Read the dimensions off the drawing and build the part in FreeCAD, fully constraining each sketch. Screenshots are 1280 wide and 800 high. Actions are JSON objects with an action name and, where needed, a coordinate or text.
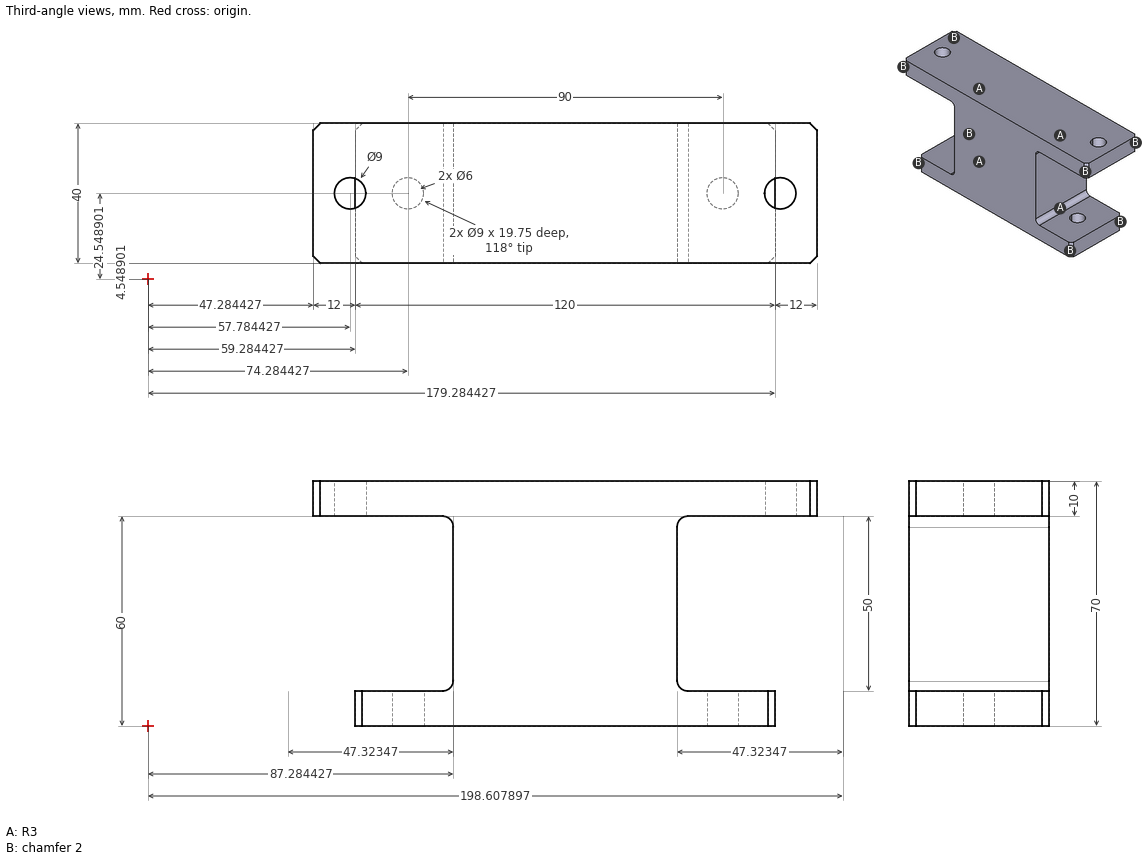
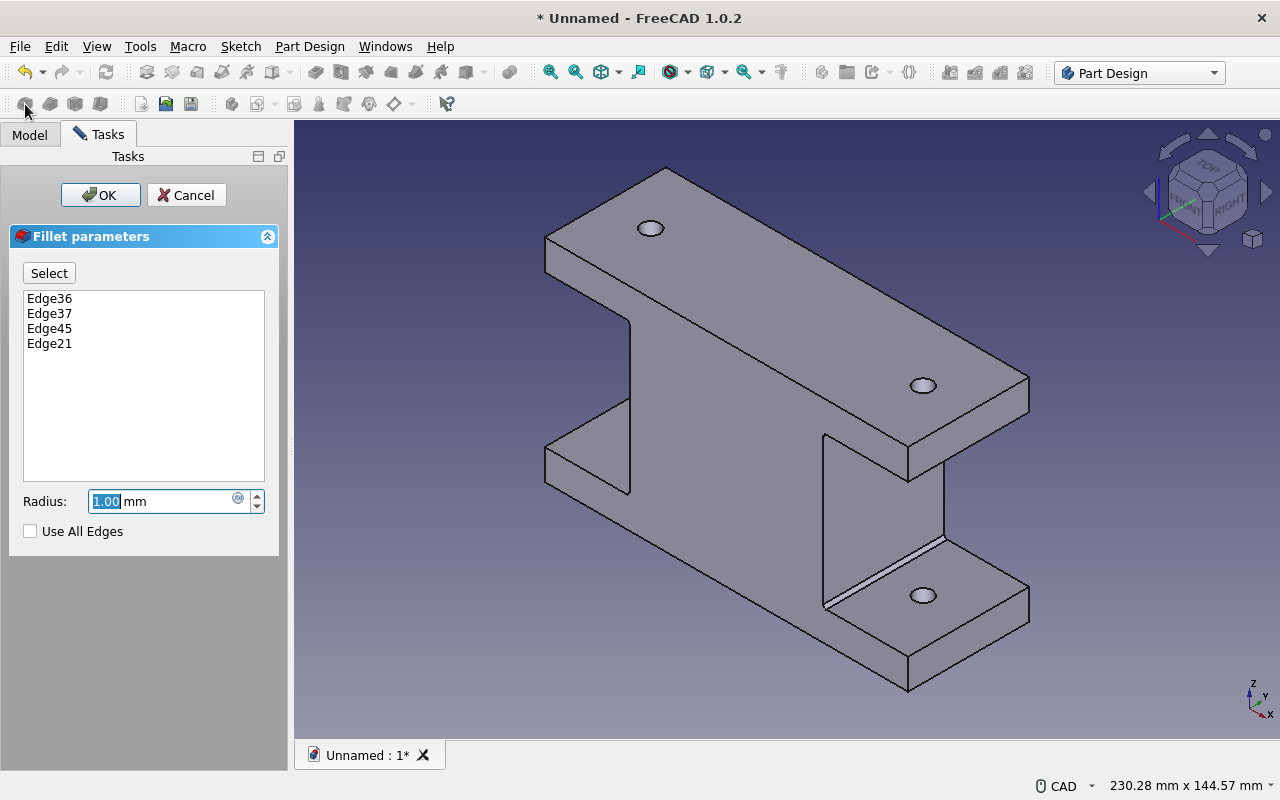
{"action": "type", "text": "3"}
{"action": "key", "text": "Tab"}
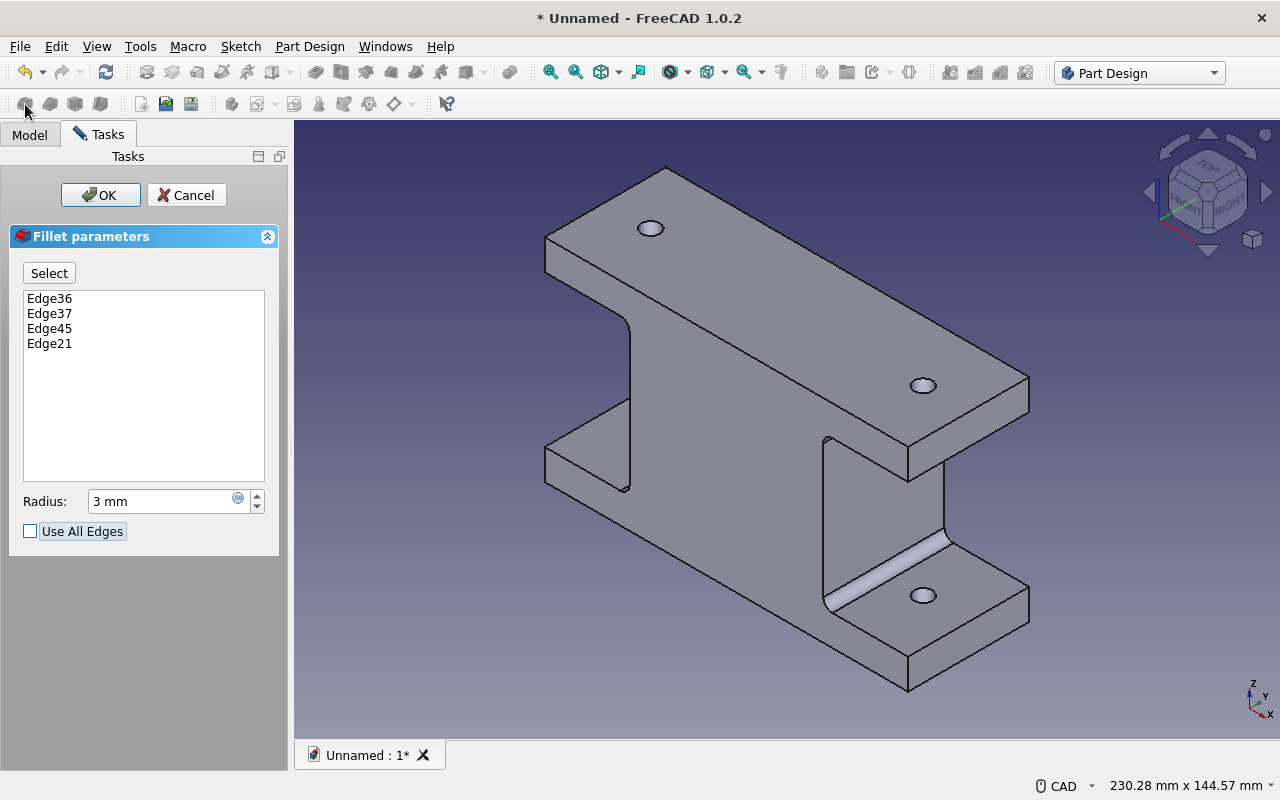
{"action": "left_click", "coordinate": [101, 195]}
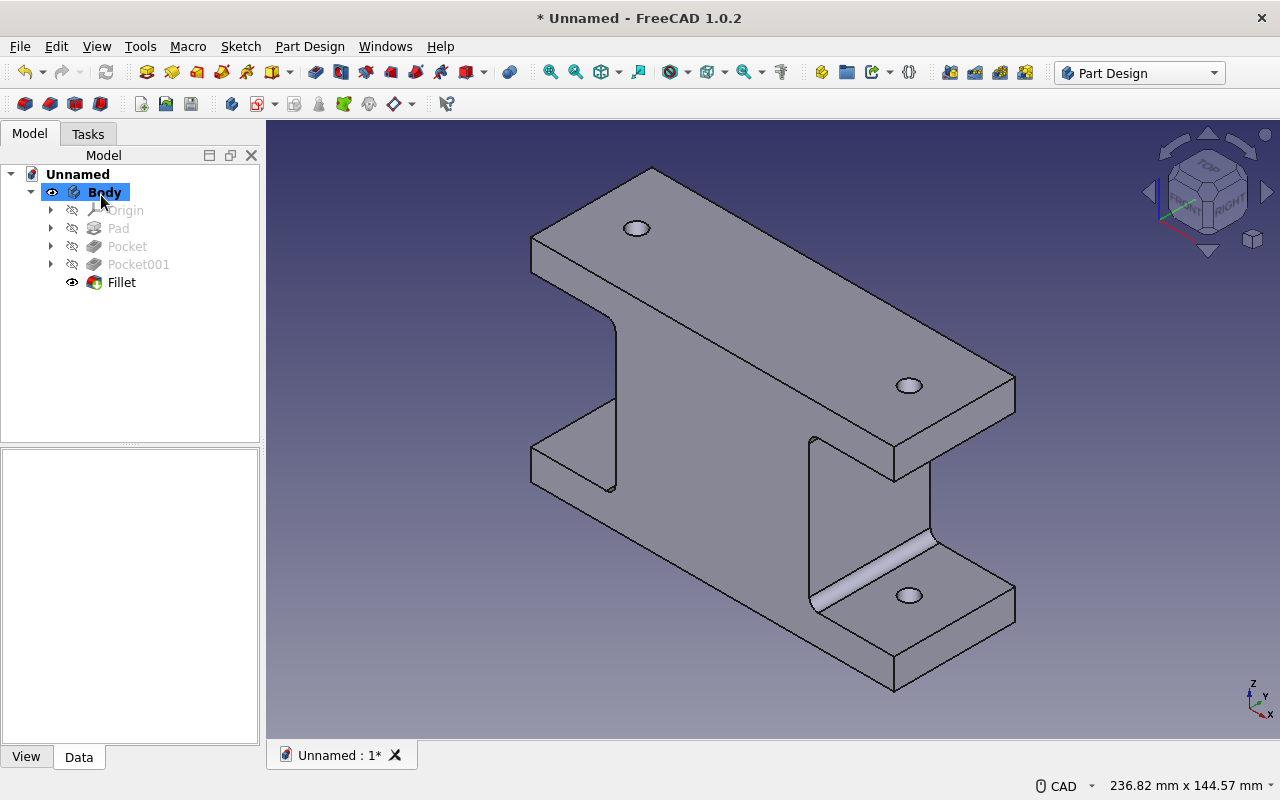
{"action": "left_click", "coordinate": [51, 210]}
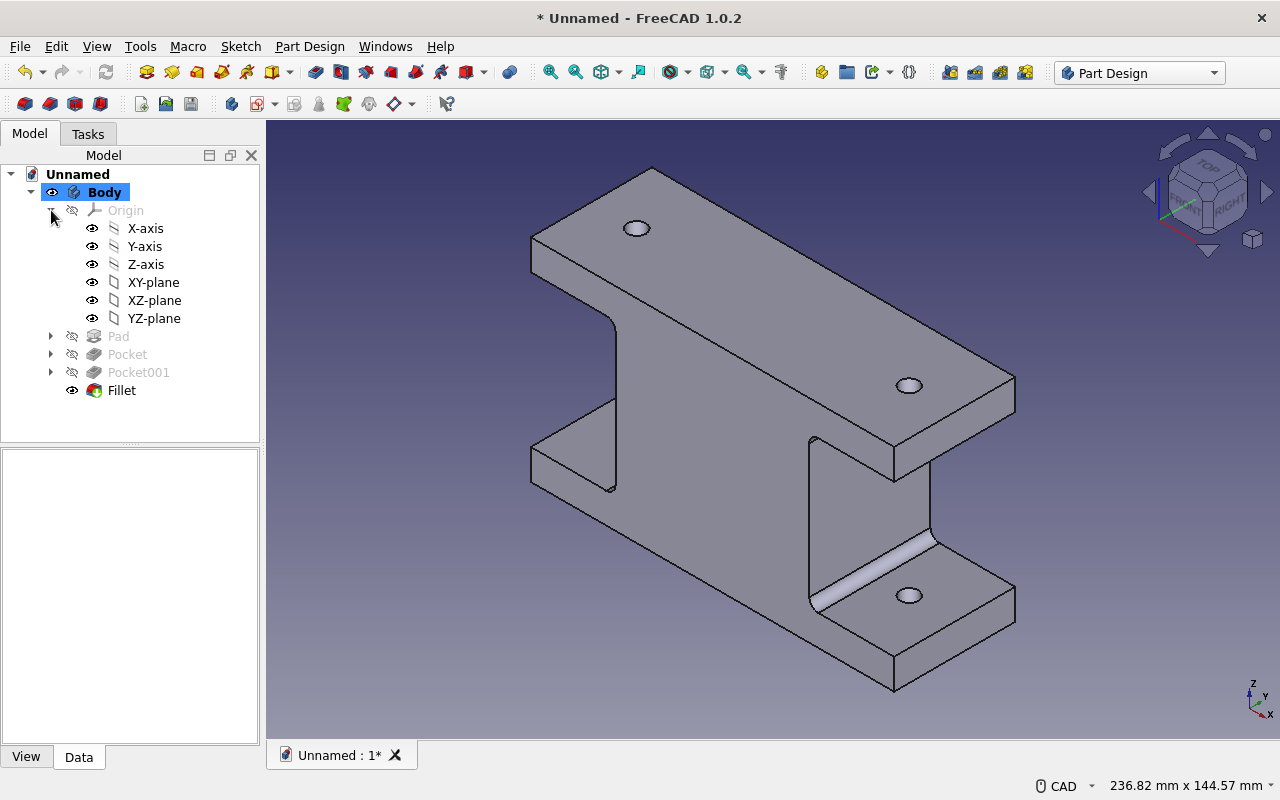
{"action": "left_click", "coordinate": [137, 282]}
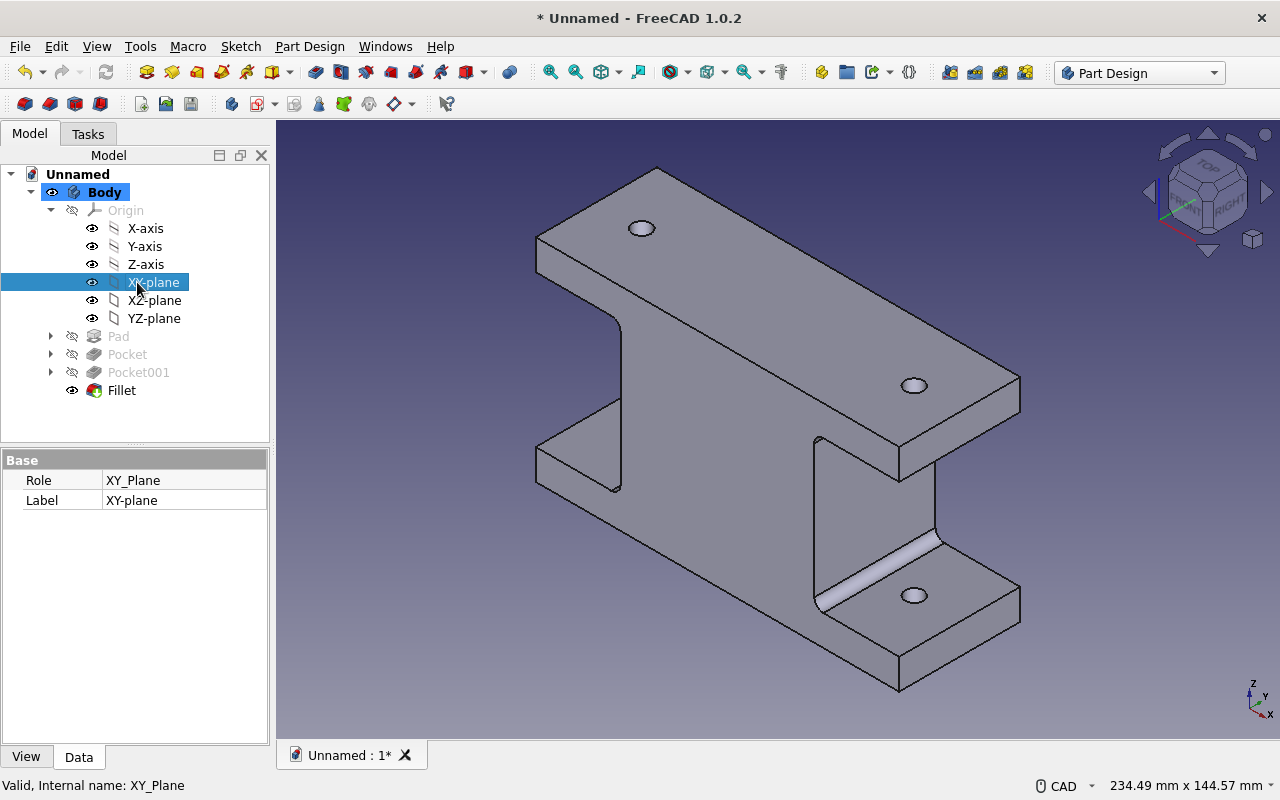
{"action": "left_click", "coordinate": [394, 104]}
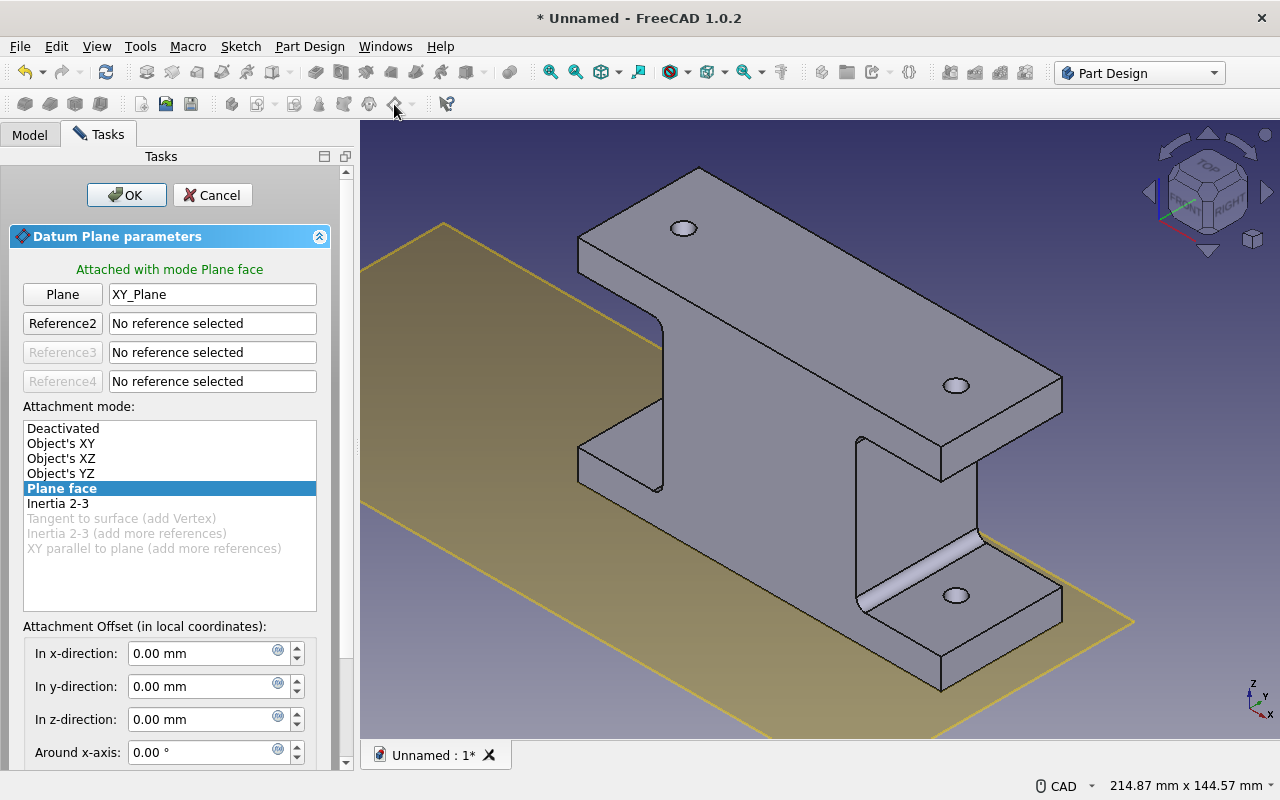
{"action": "triple_click", "coordinate": [210, 720]}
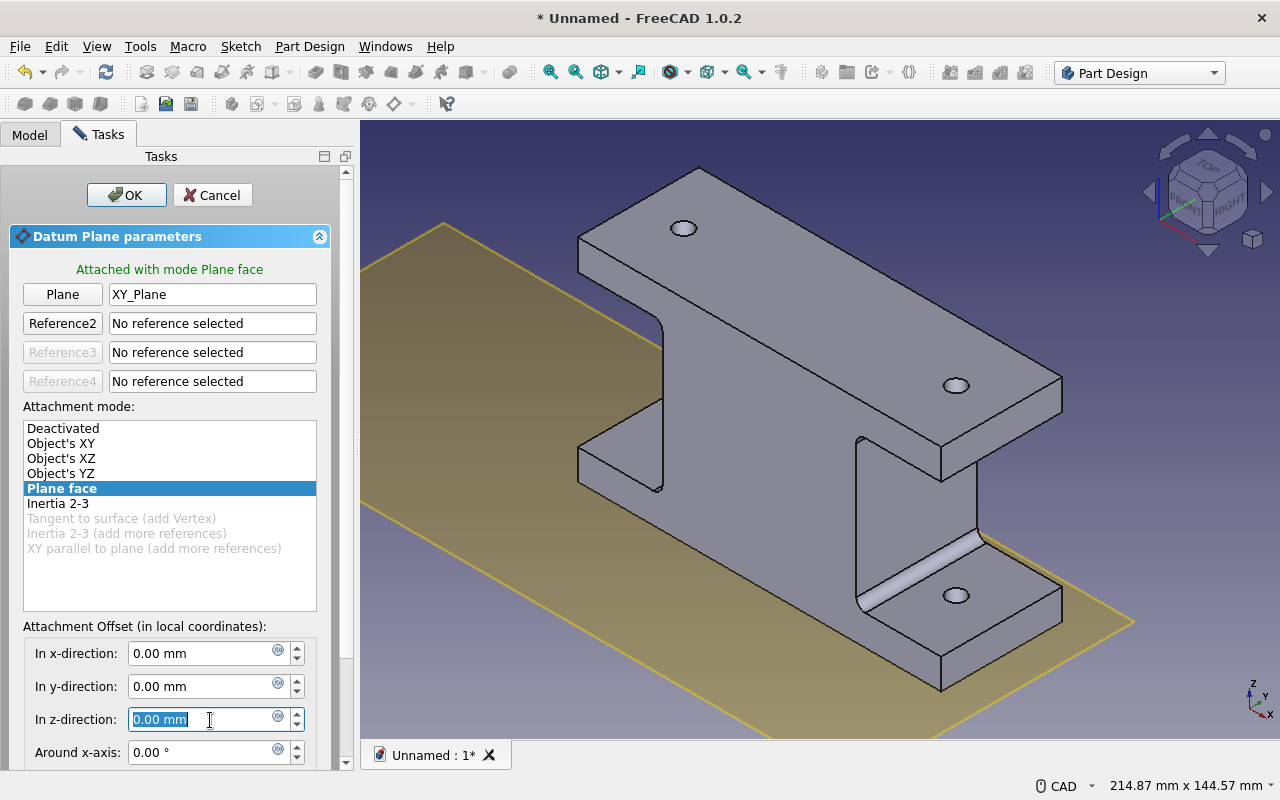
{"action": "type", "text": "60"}
{"action": "key", "text": "Tab"}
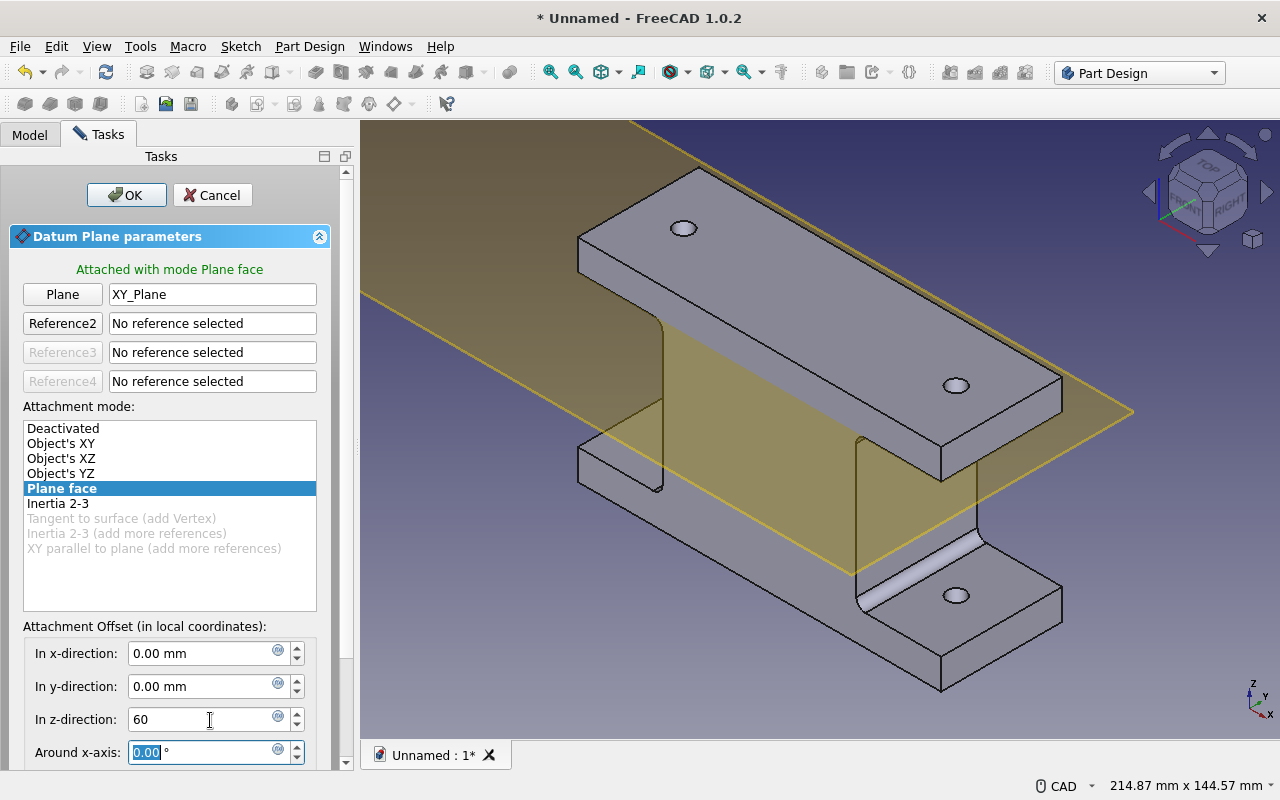
{"action": "left_click", "coordinate": [127, 195]}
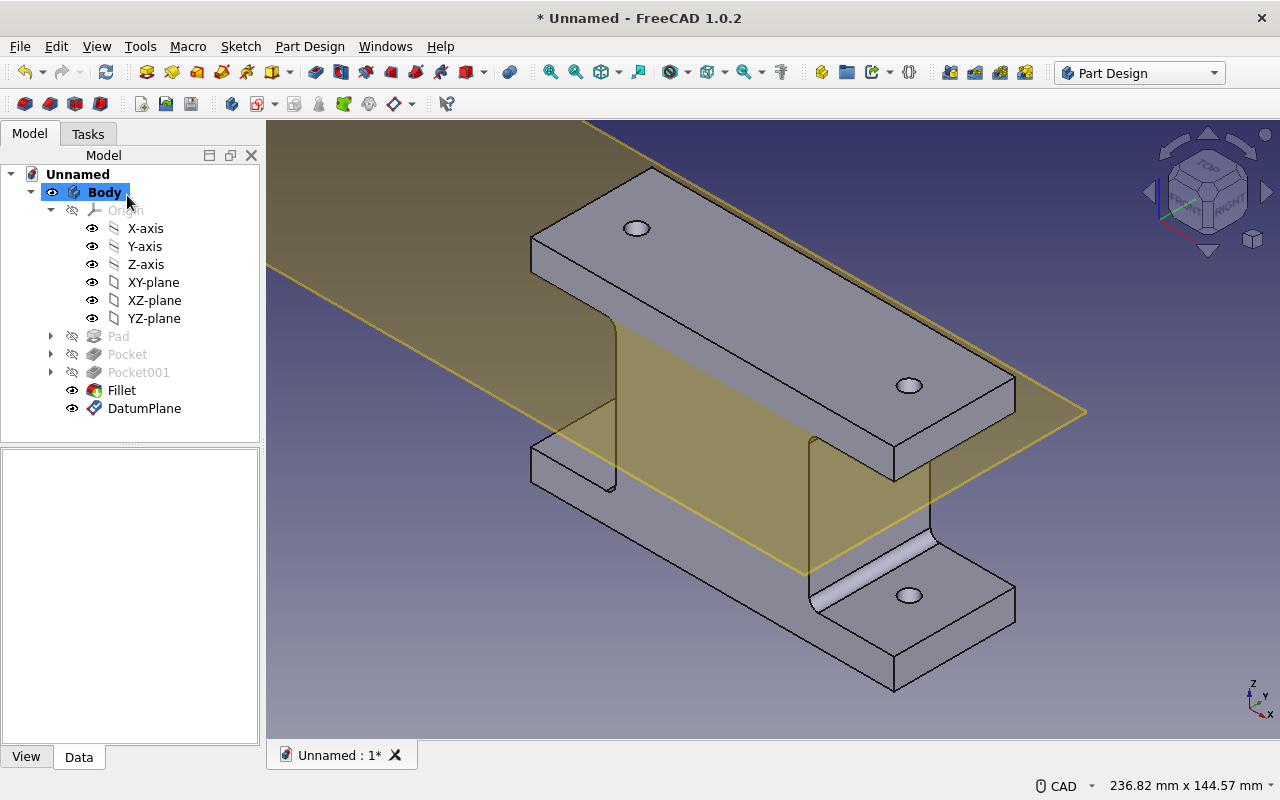
{"action": "left_click", "coordinate": [117, 408]}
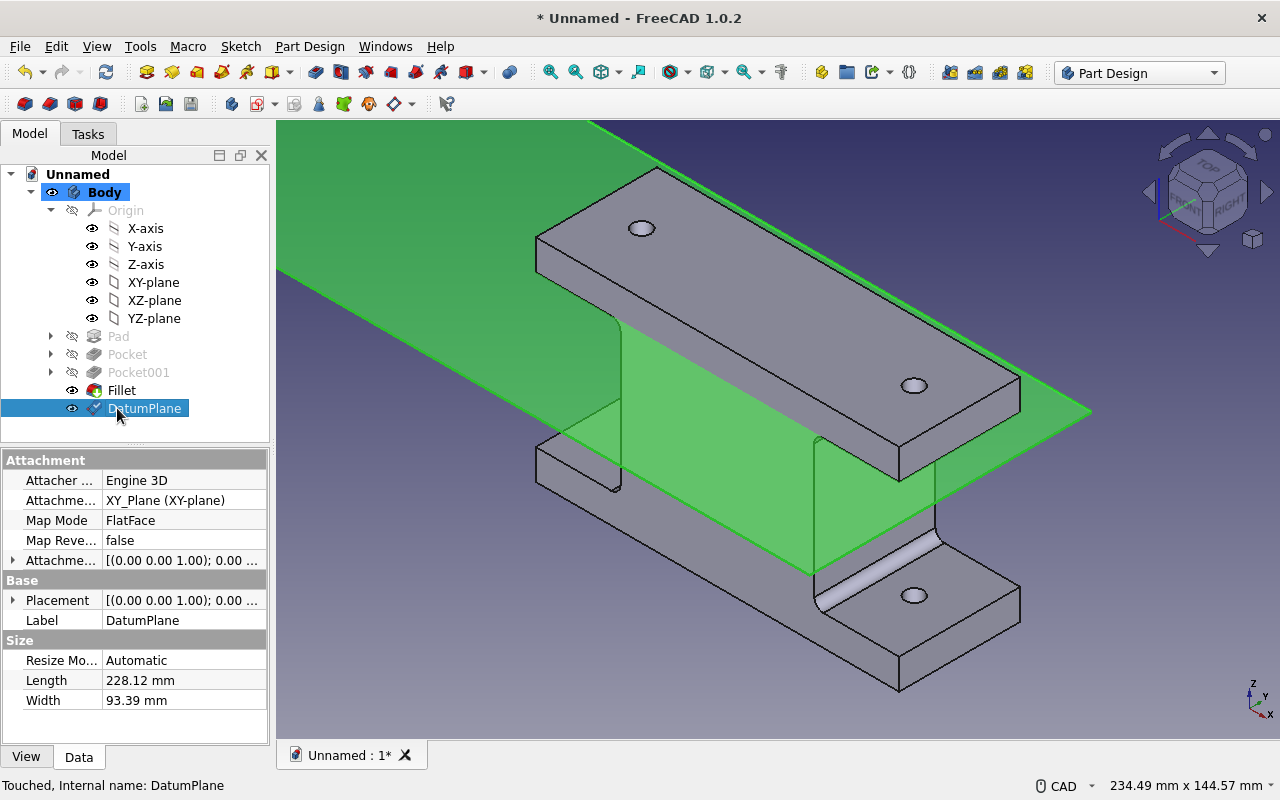
{"action": "left_click", "coordinate": [256, 104]}